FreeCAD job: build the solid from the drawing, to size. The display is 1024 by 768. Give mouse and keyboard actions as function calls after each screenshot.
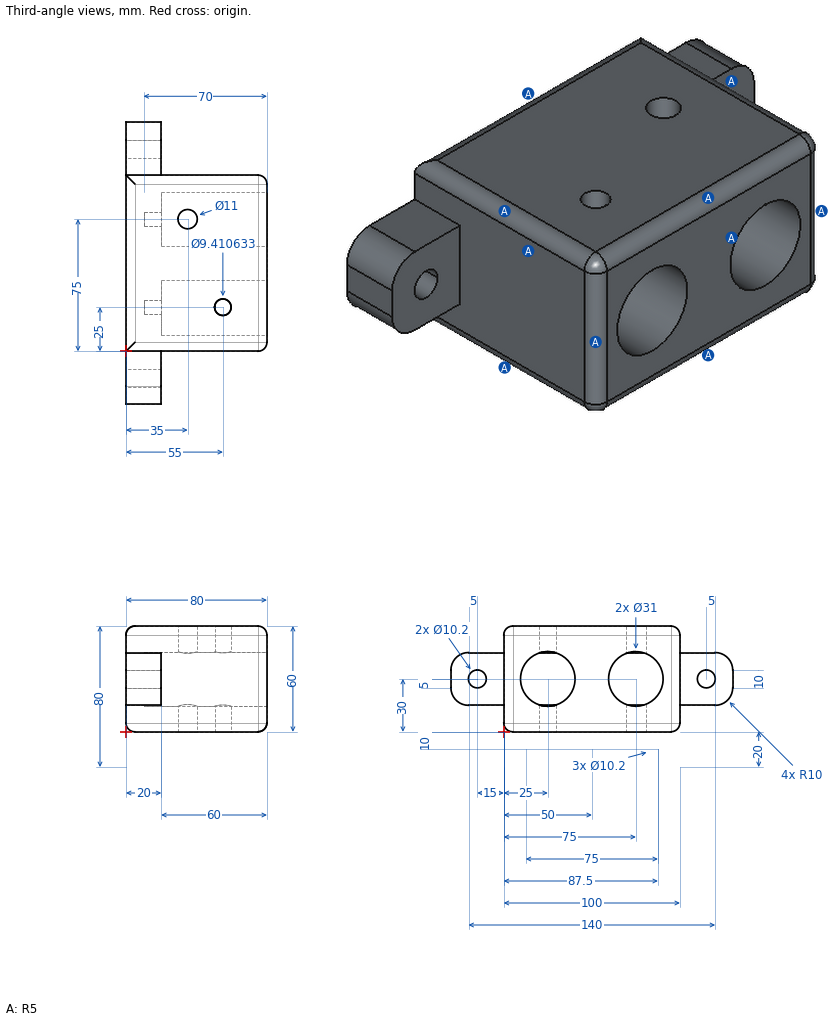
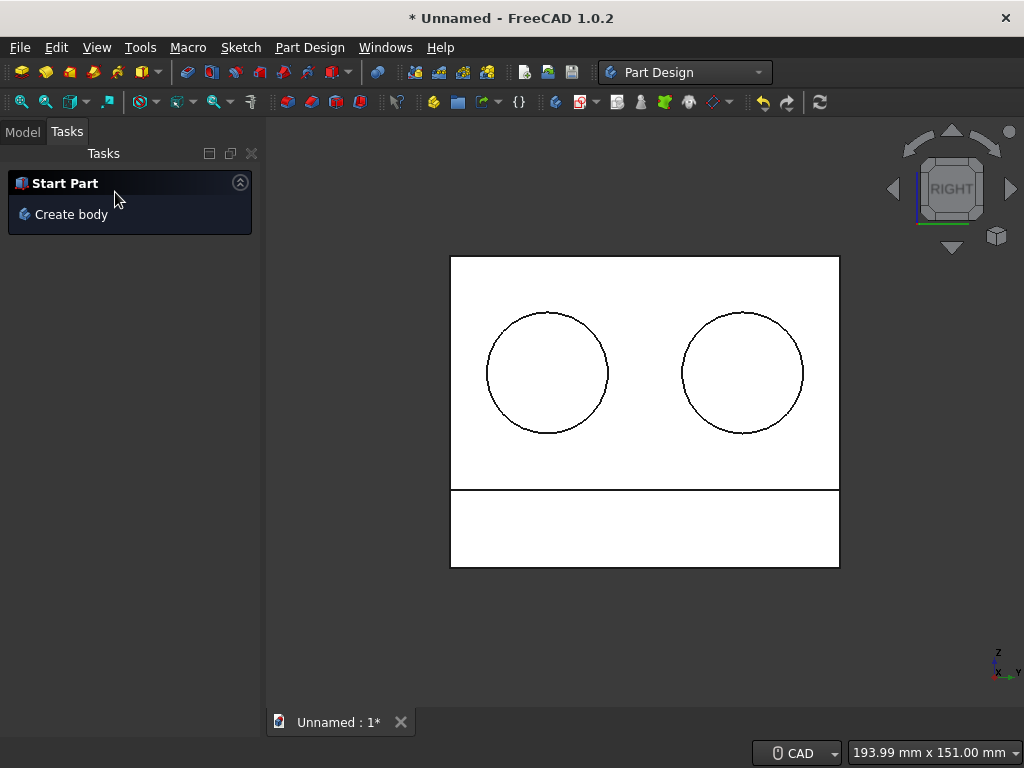
click(757, 528)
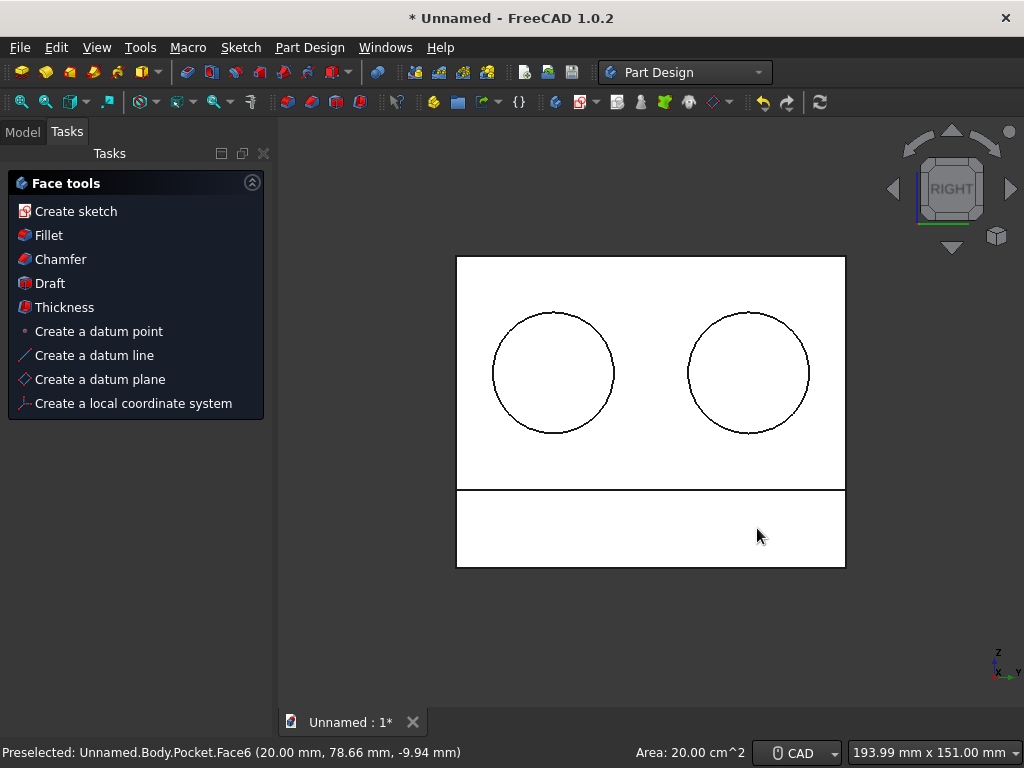
click(580, 102)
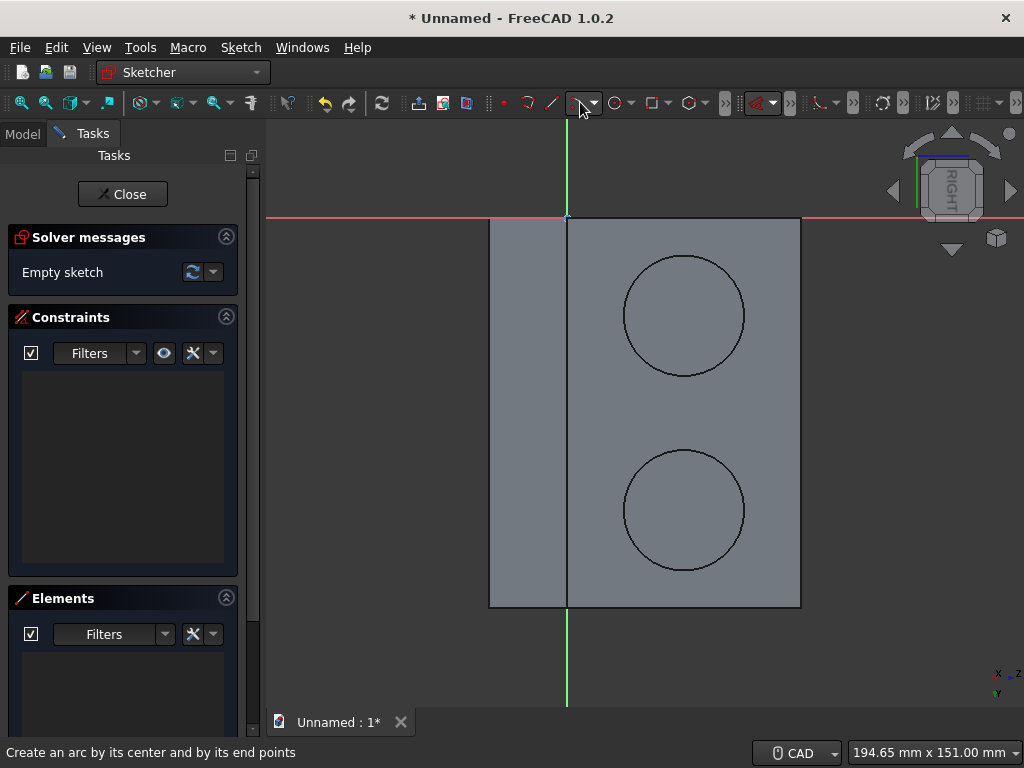
key(g)
key(c)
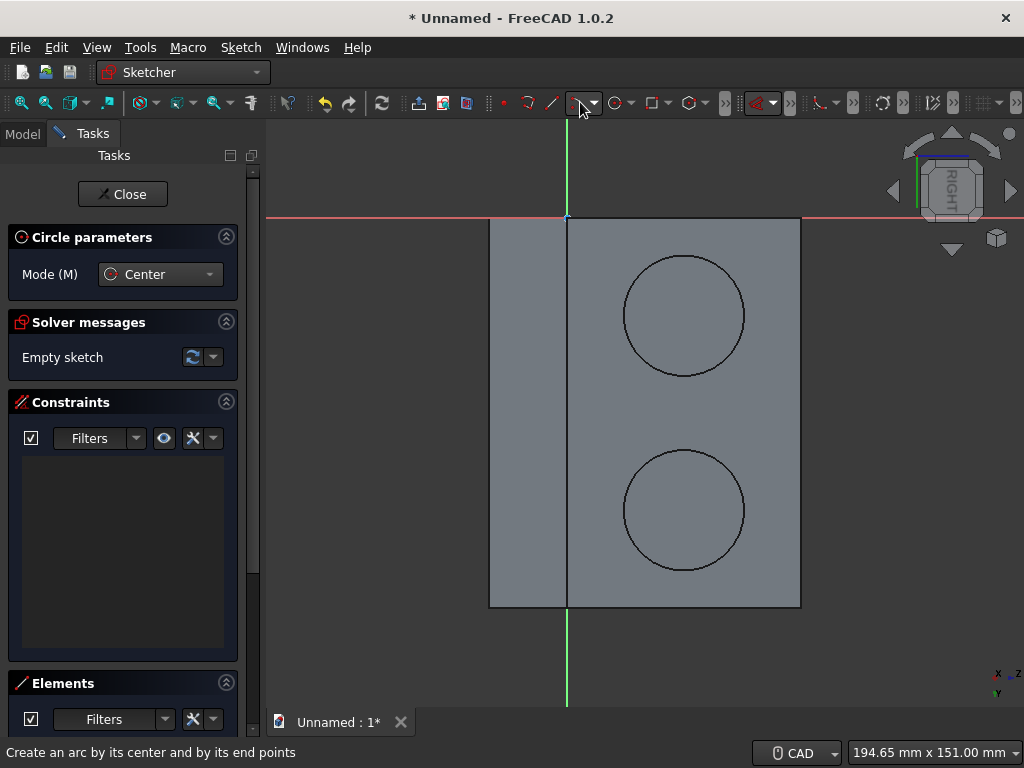
click(528, 559)
move(542, 545)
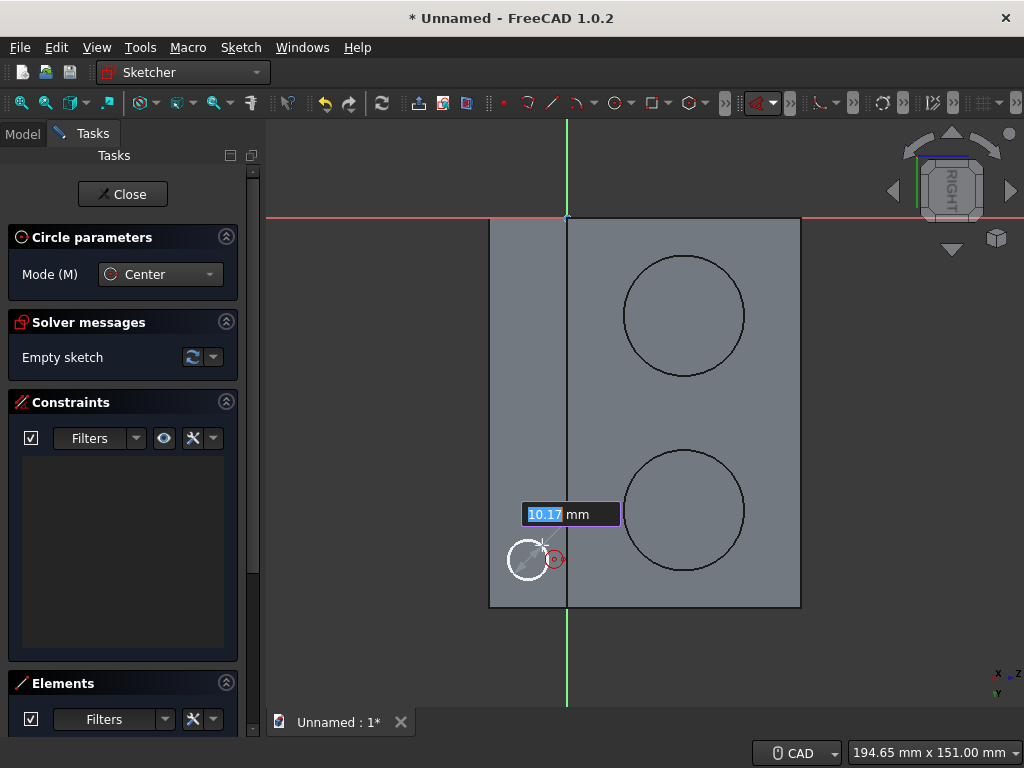
text(10.2)
key(Return)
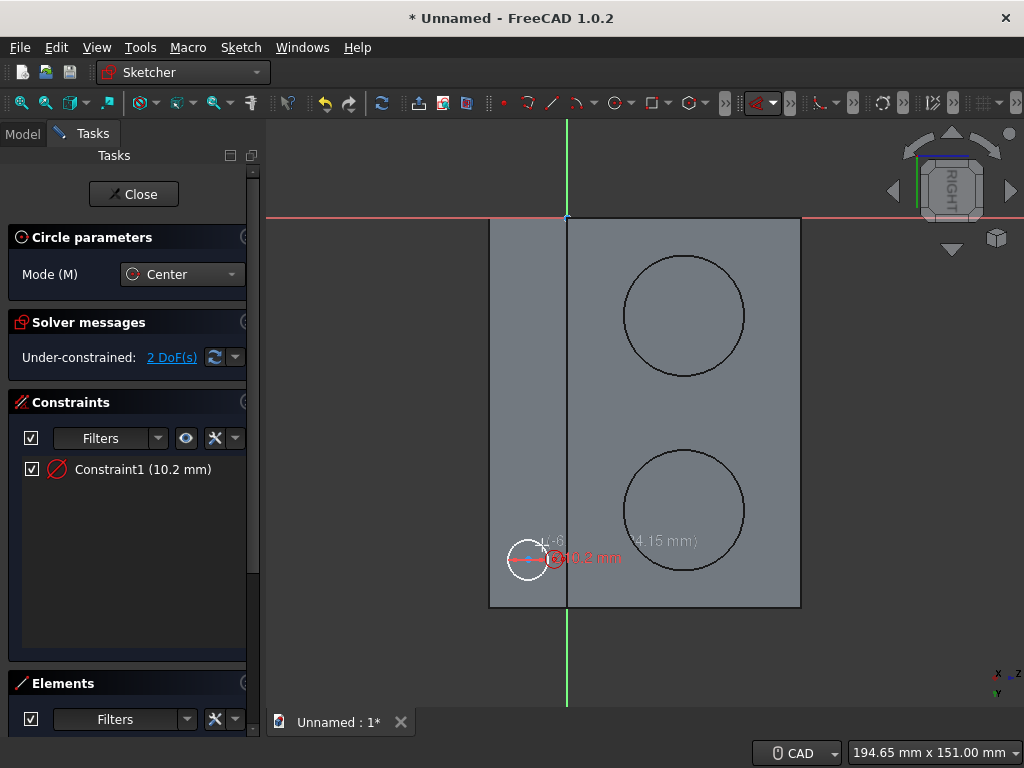
click(528, 267)
move(542, 253)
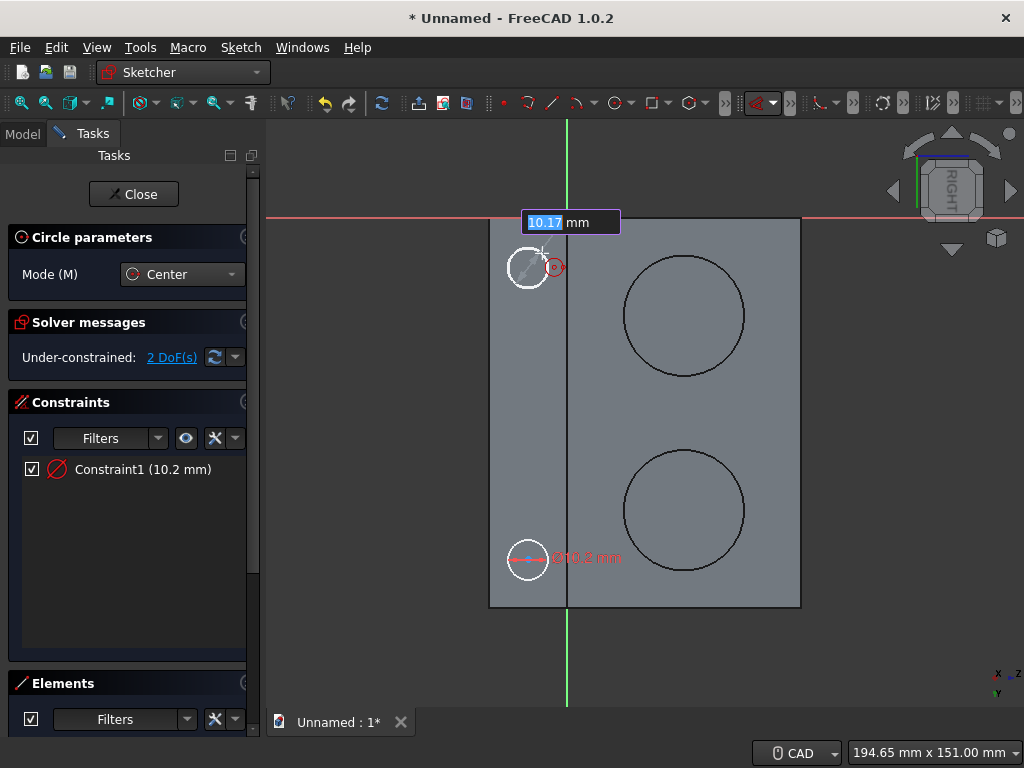
text(10.2)
key(Return)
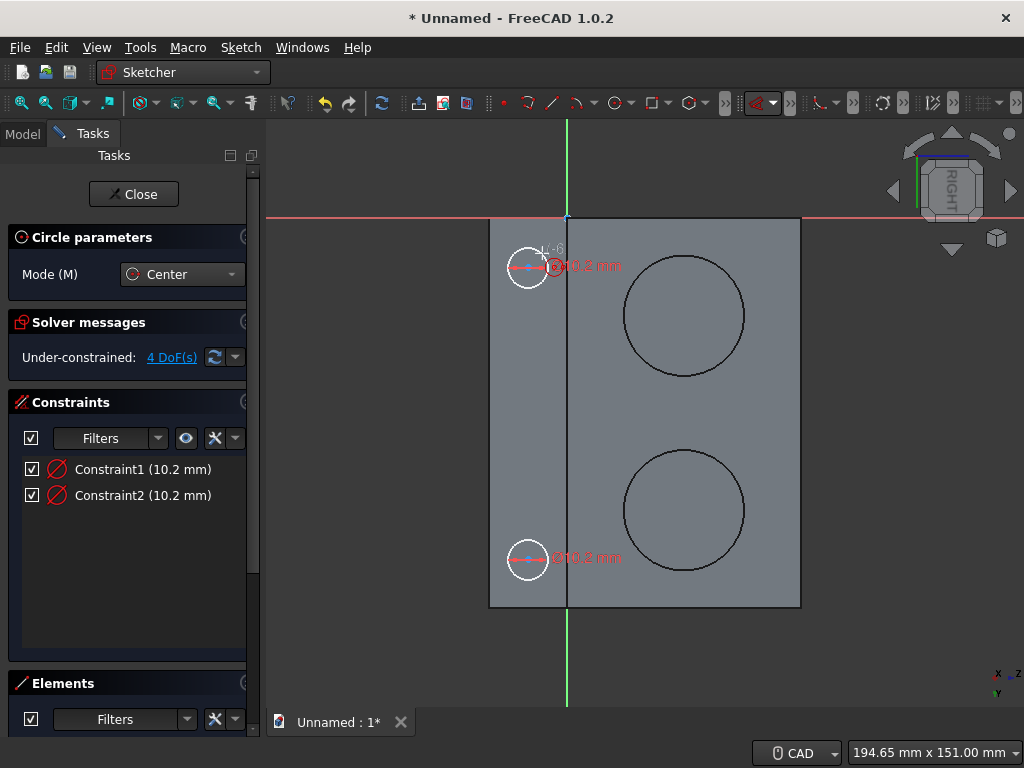
click(528, 413)
move(542, 399)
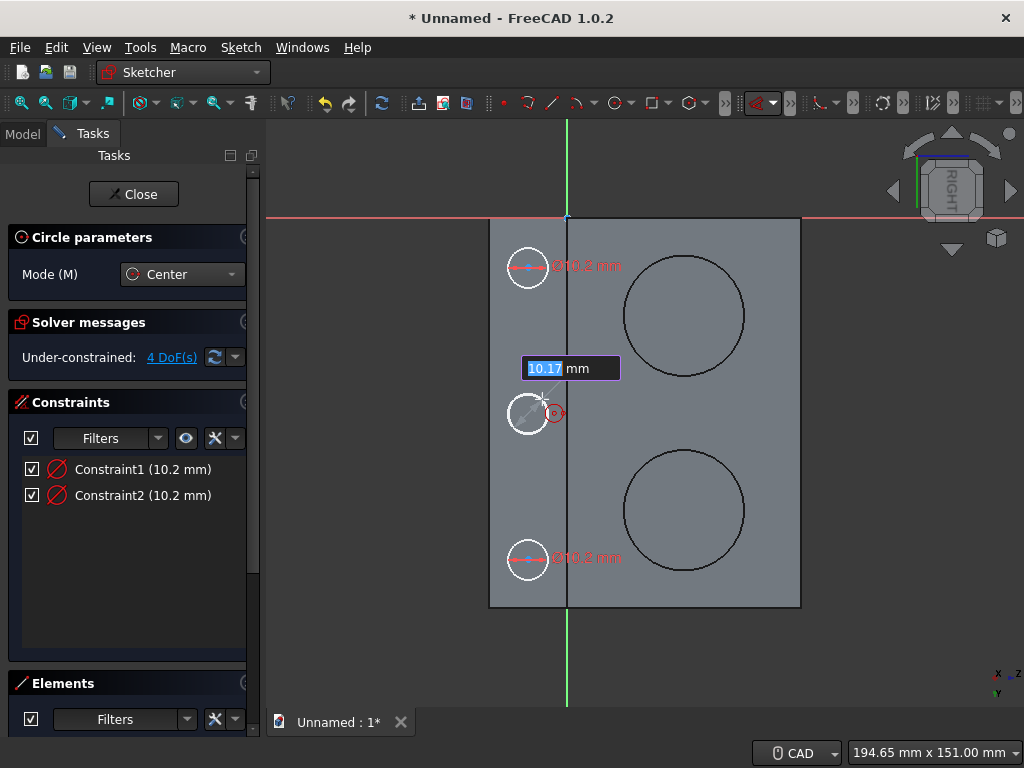
text(10.2)
key(Return)
key(Escape)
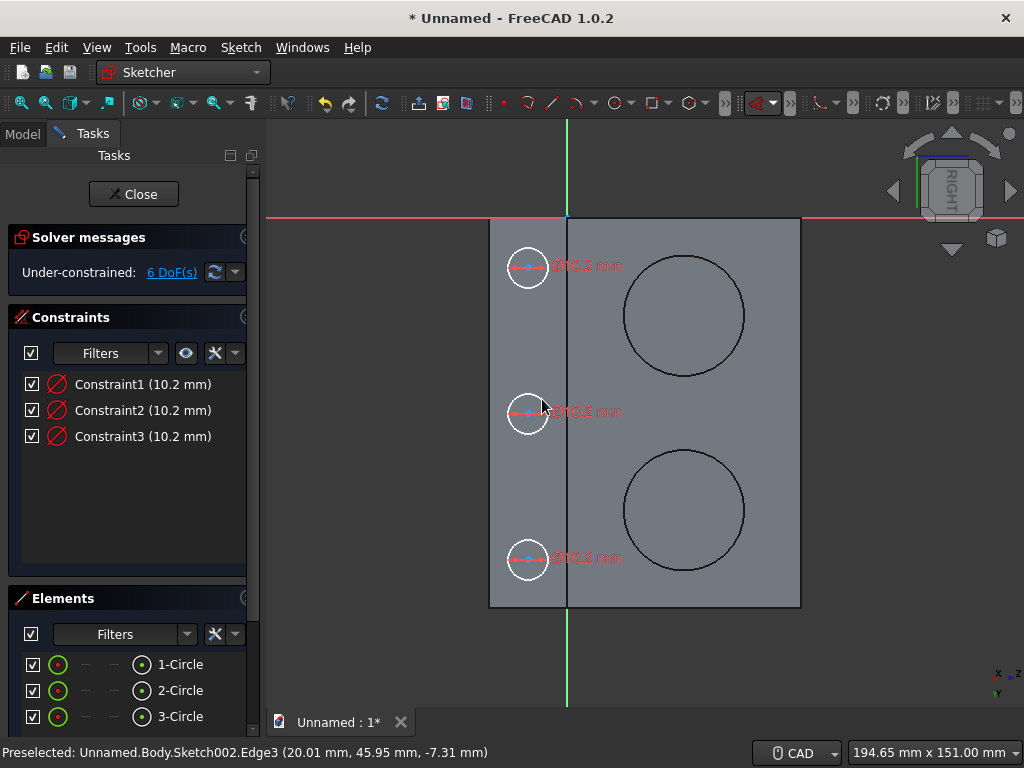
click(528, 560)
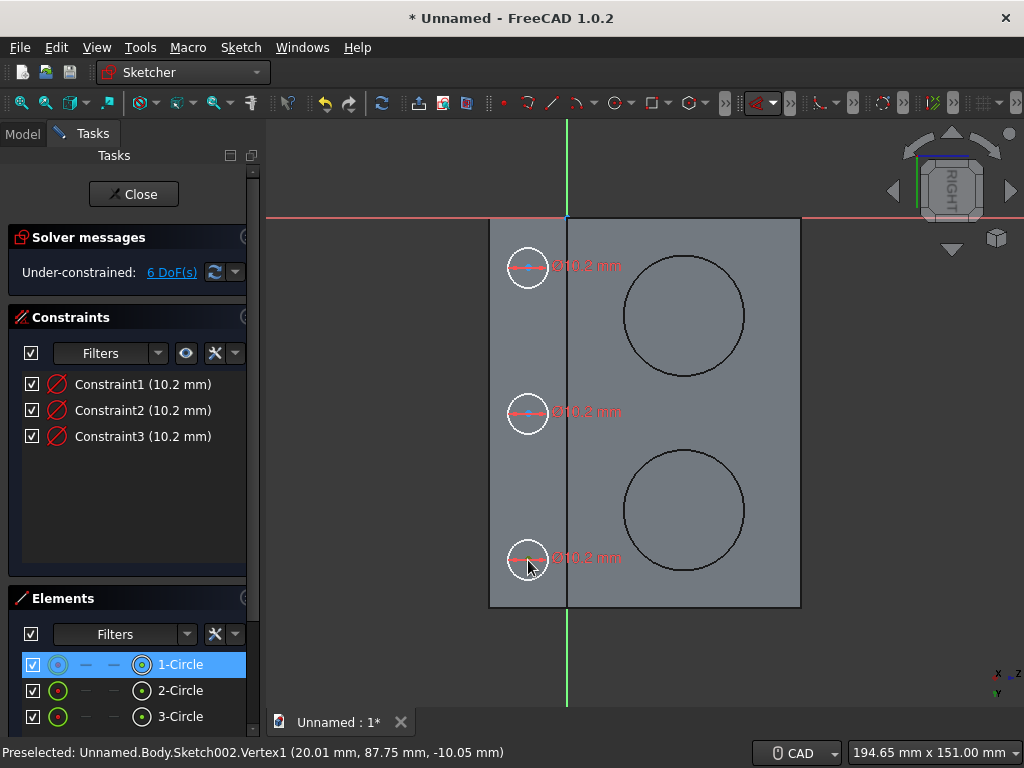
click(528, 268)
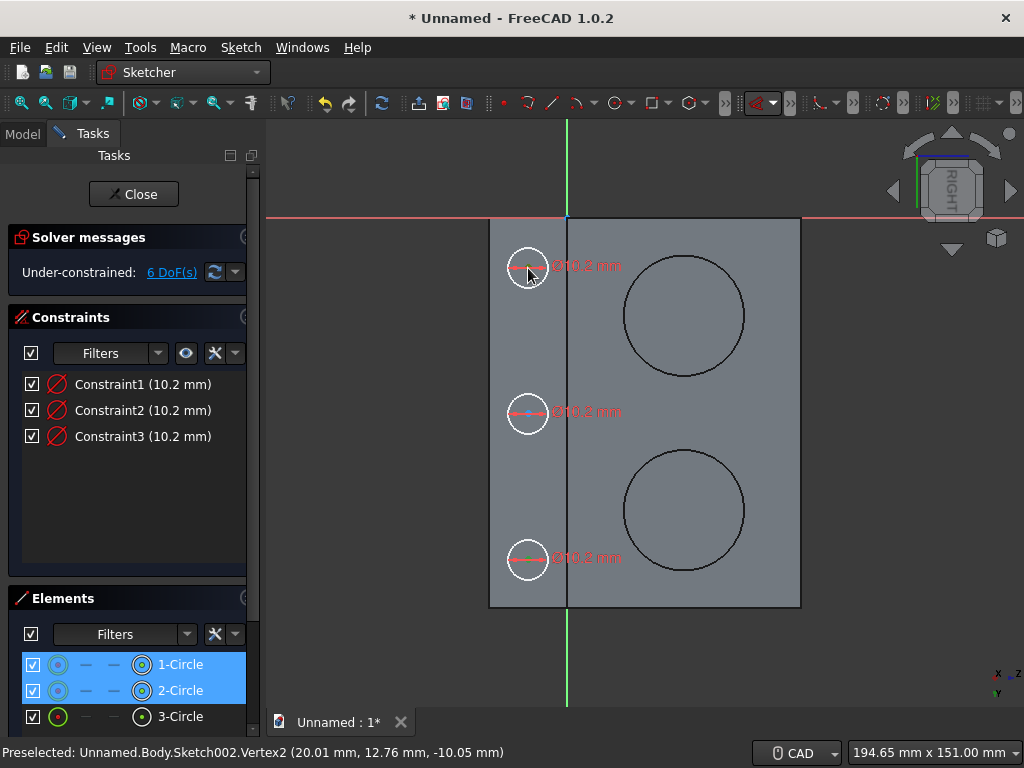
key(v)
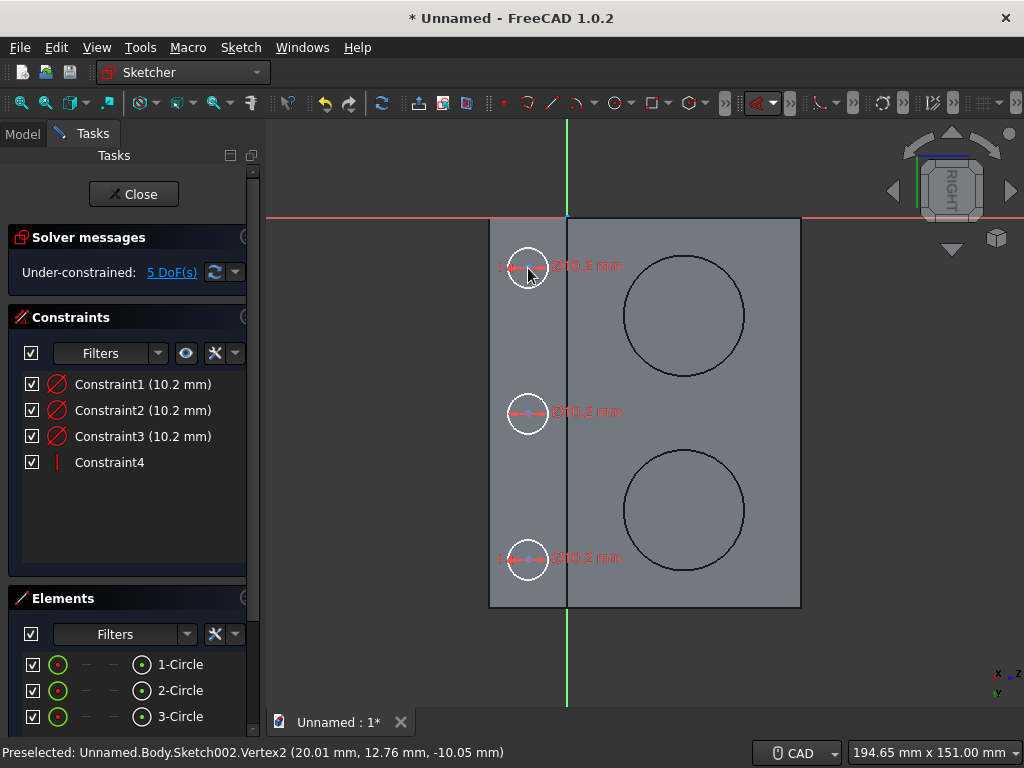
click(528, 560)